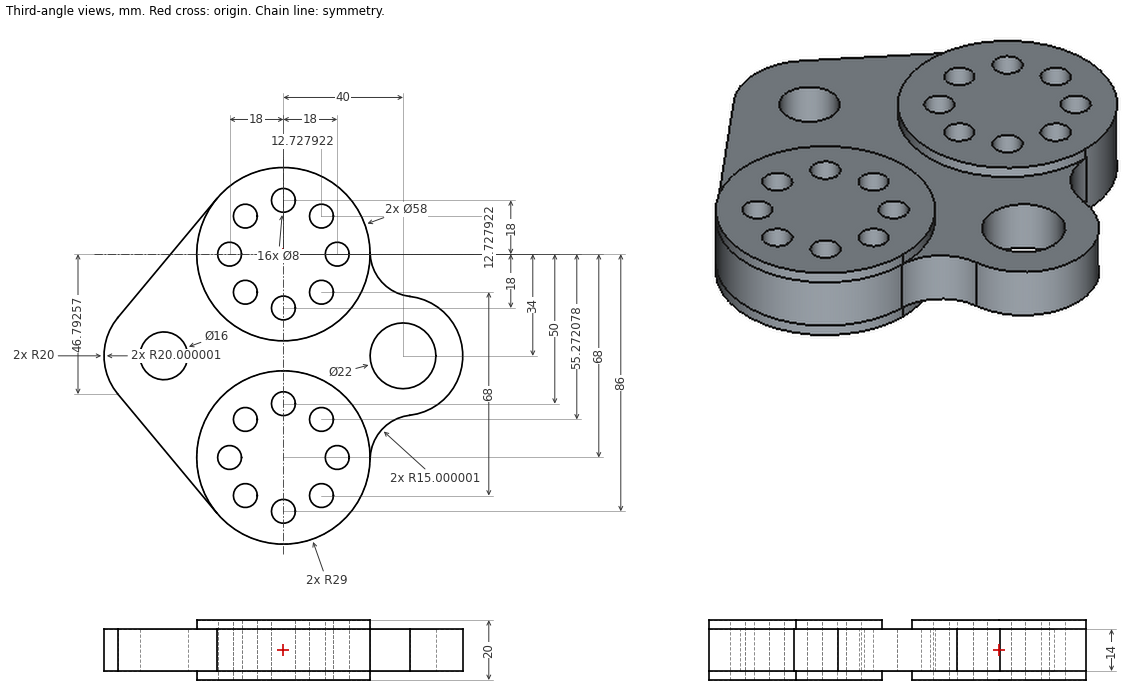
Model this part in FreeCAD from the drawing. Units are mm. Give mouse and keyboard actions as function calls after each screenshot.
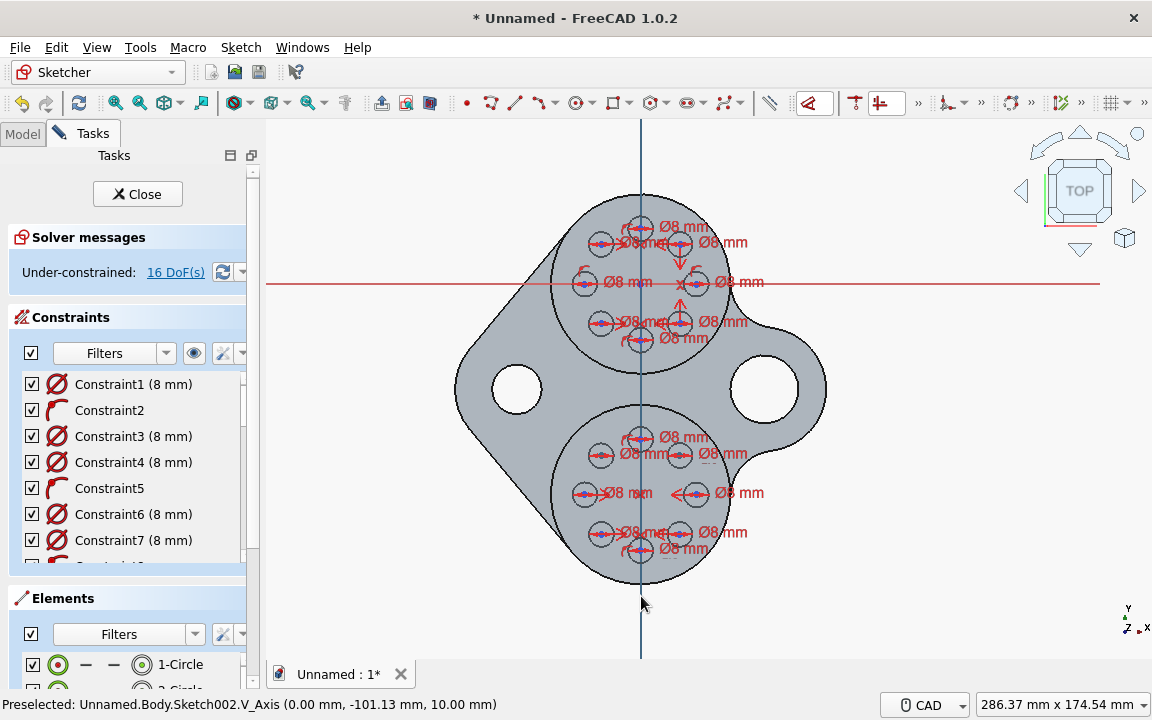
key(s)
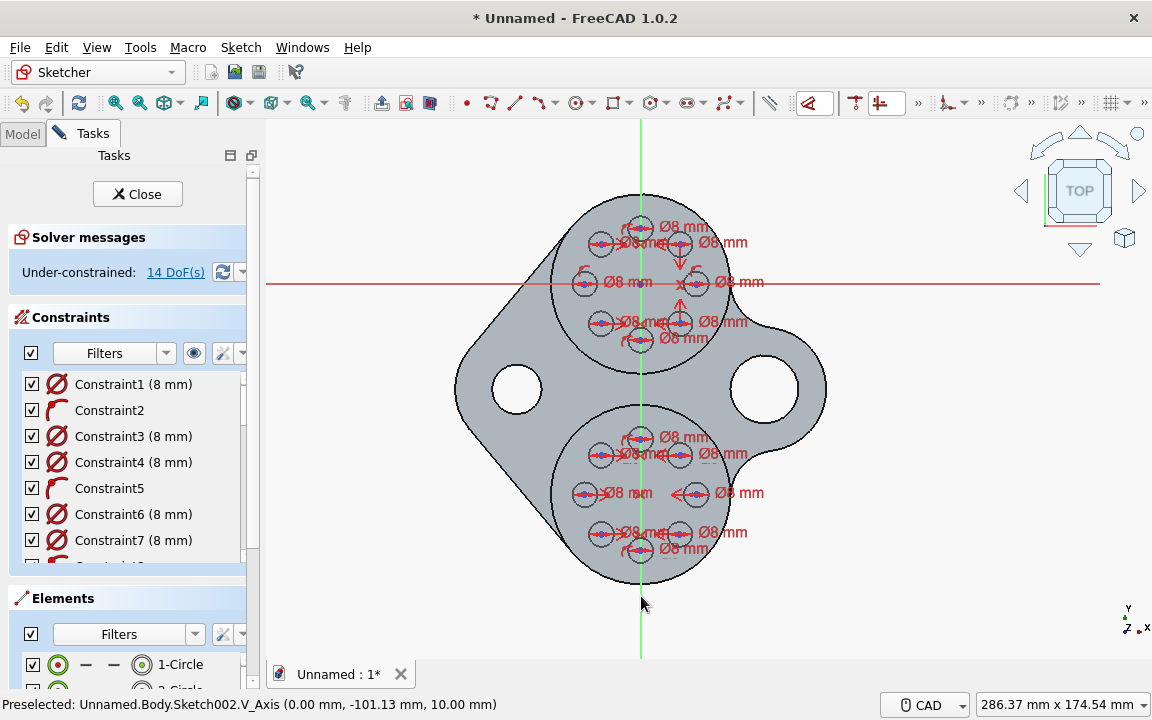
click(641, 229)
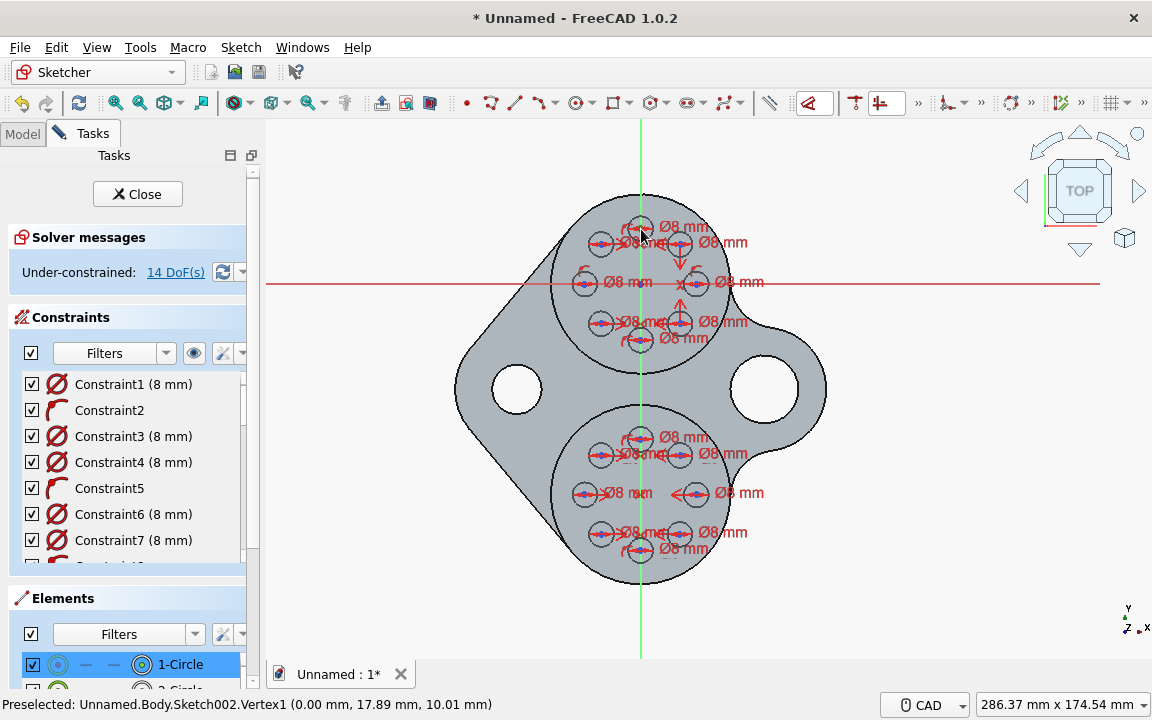
key(i)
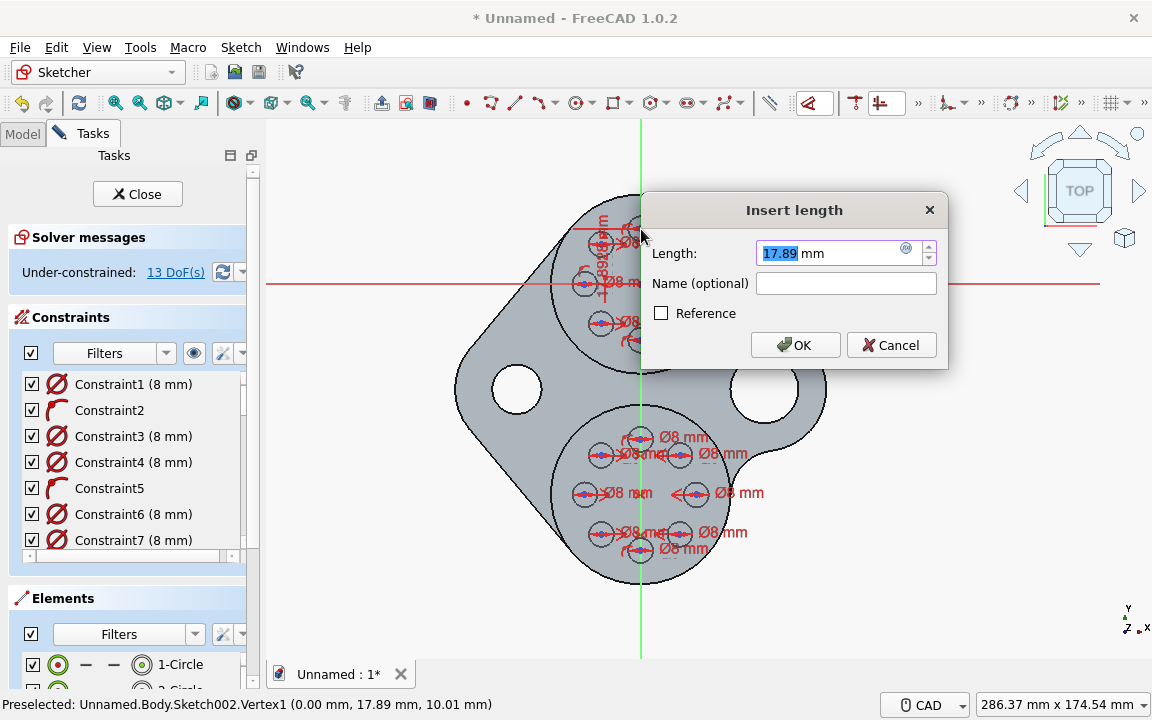
text(18)
key(Return)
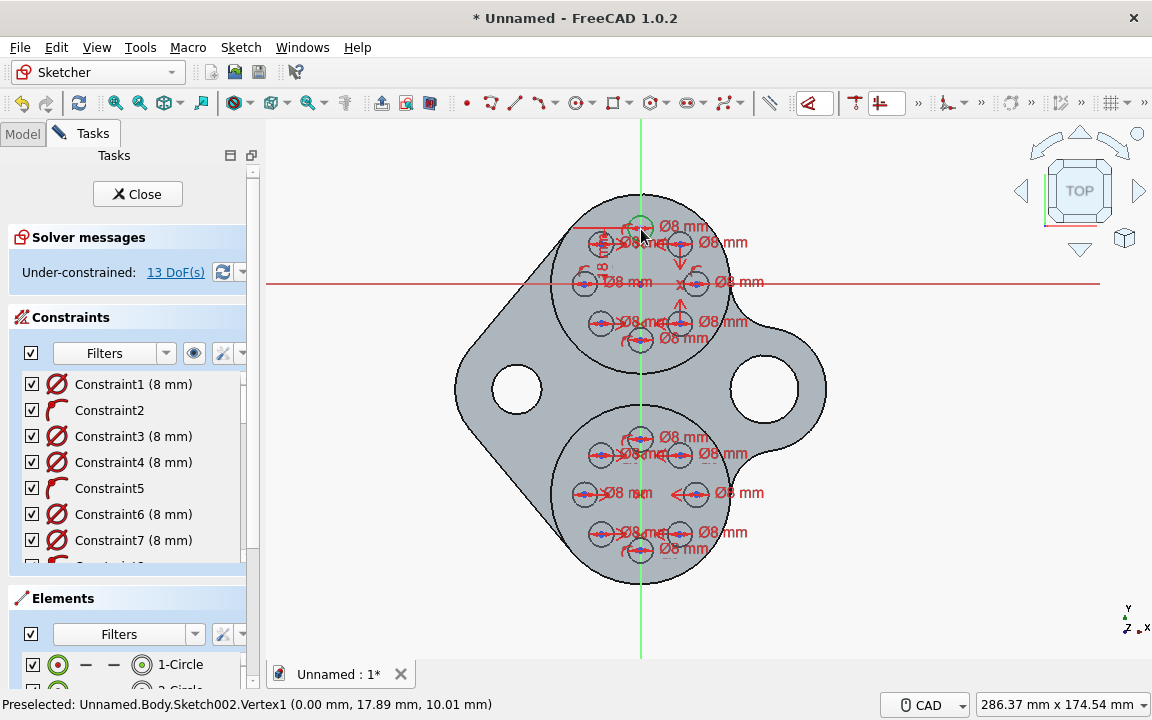
click(696, 284)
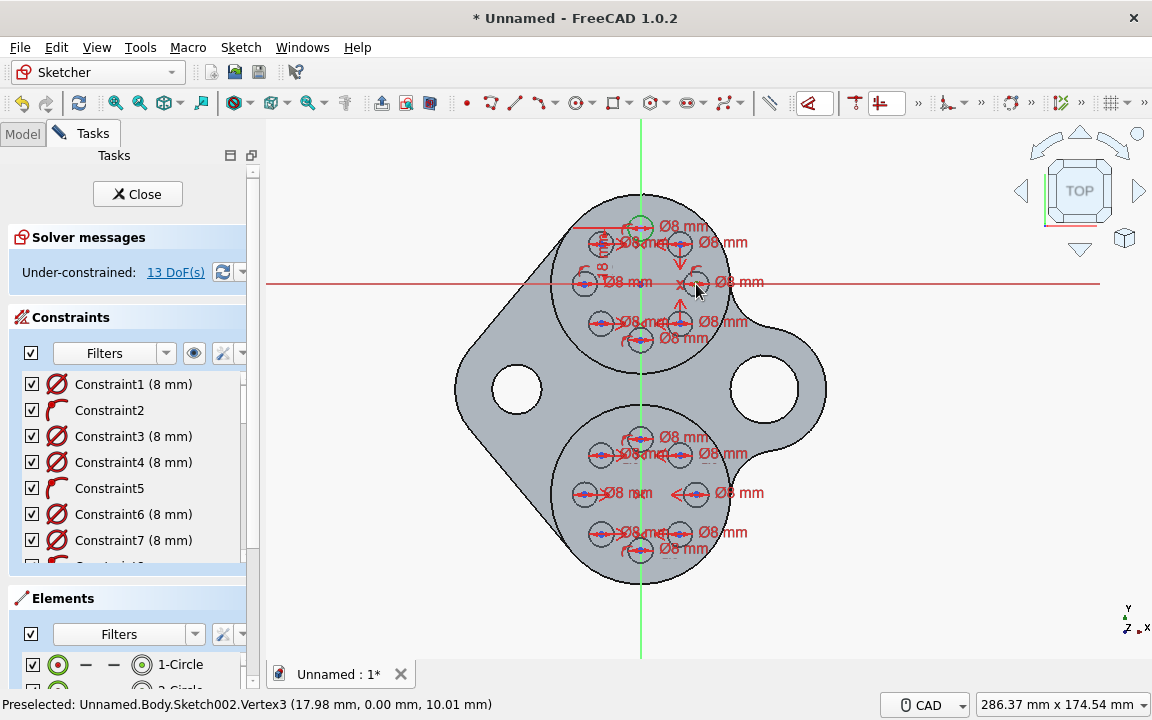
key(l)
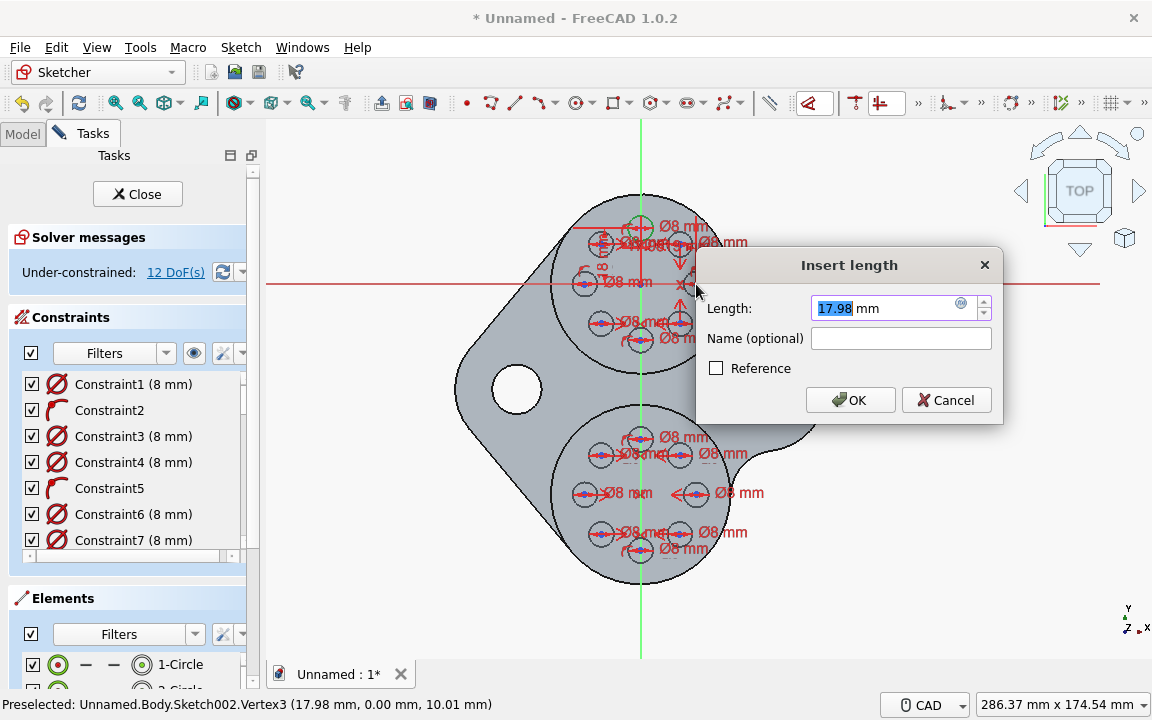
text(18)
key(Return)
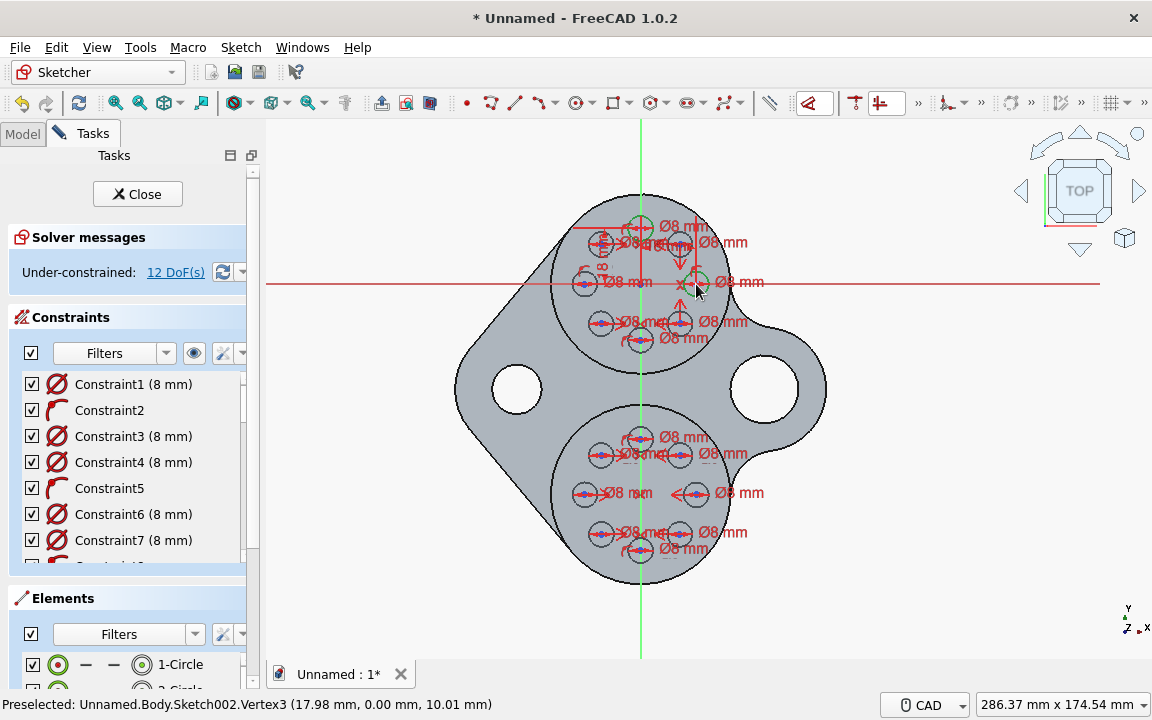
click(641, 340)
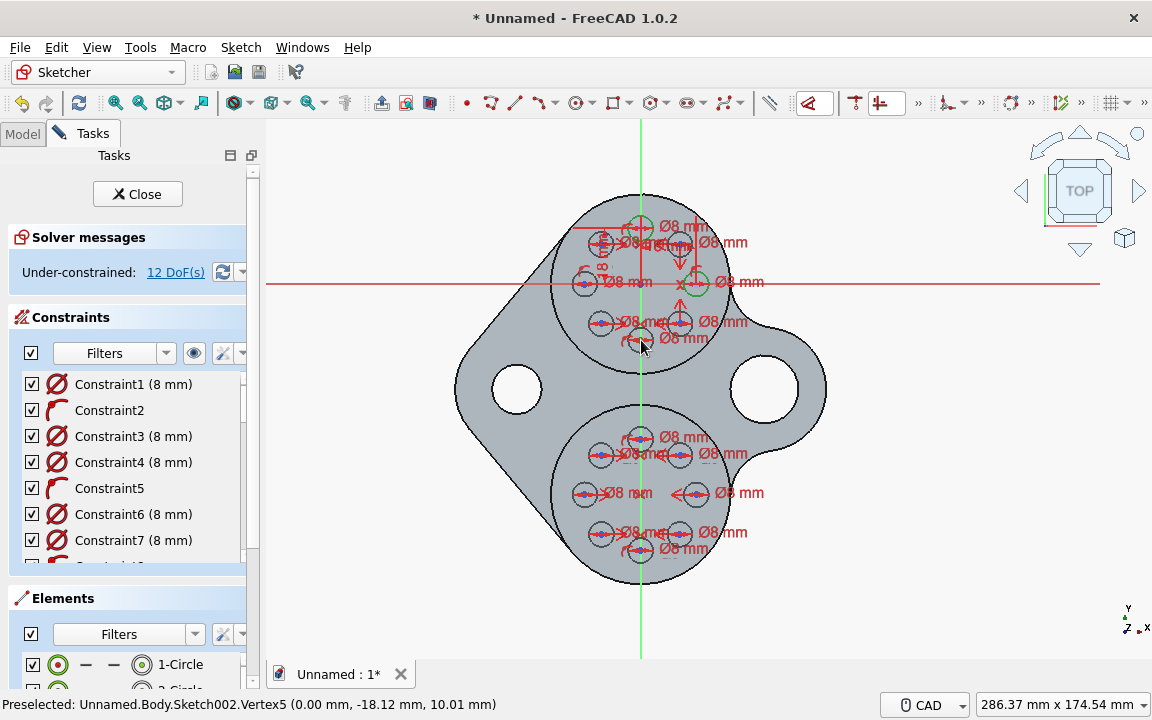
key(i)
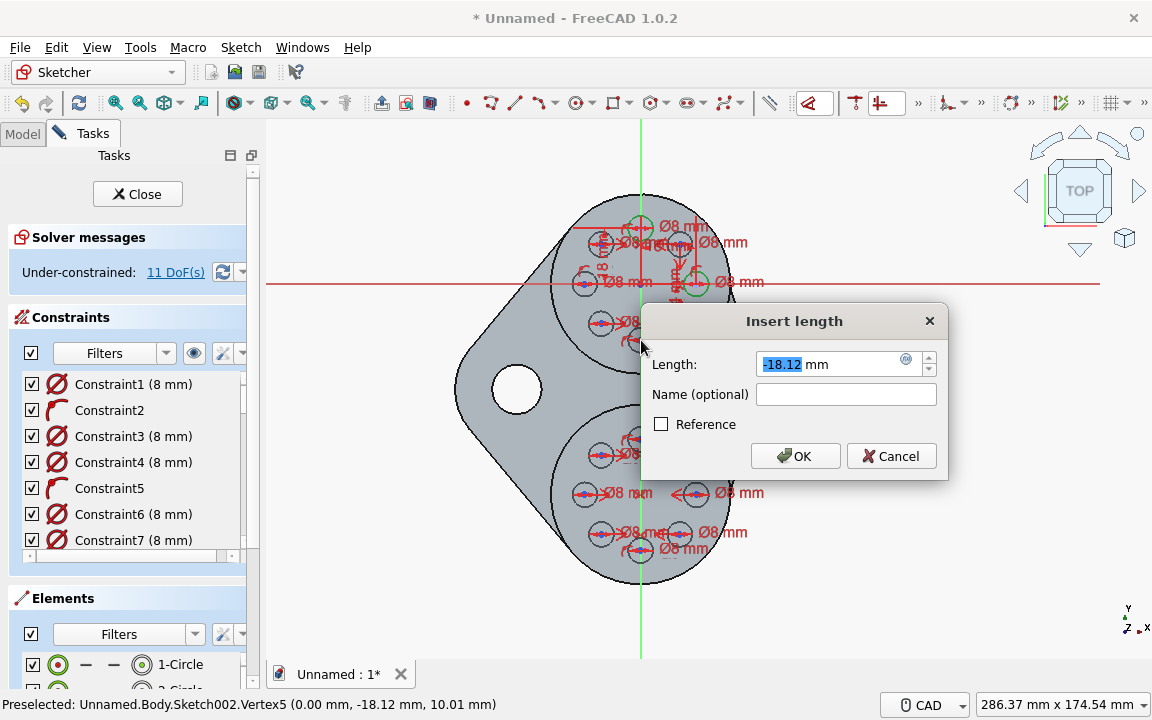
text(-18)
key(Return)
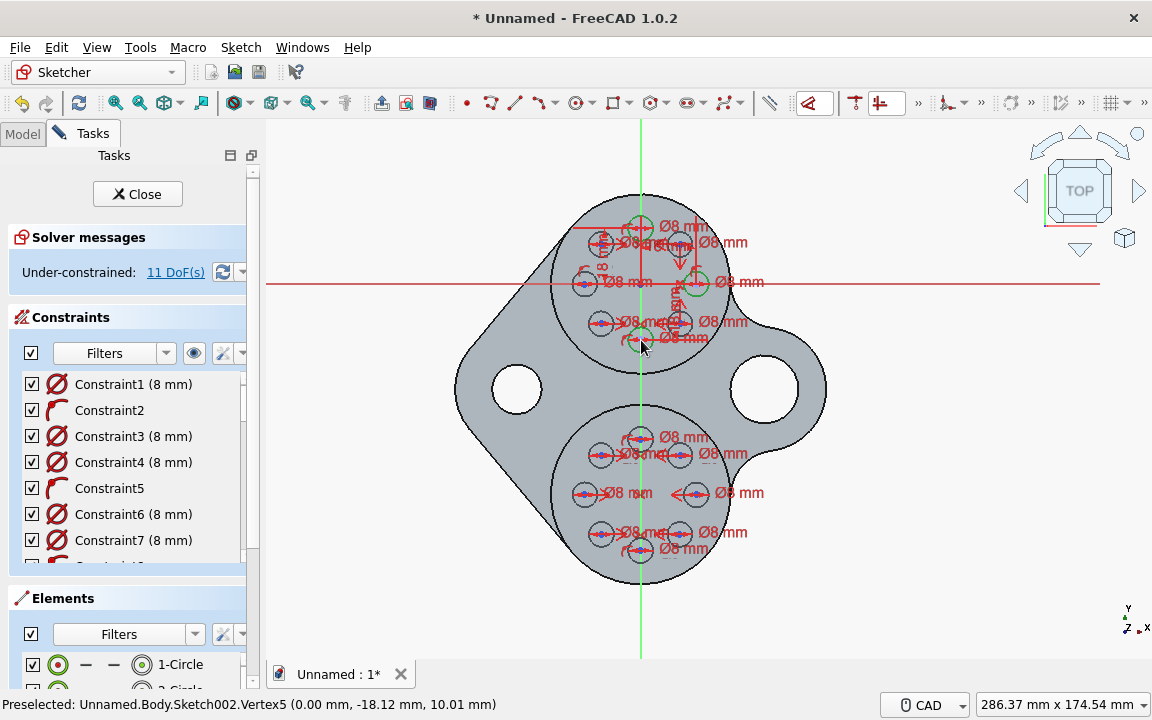
click(585, 284)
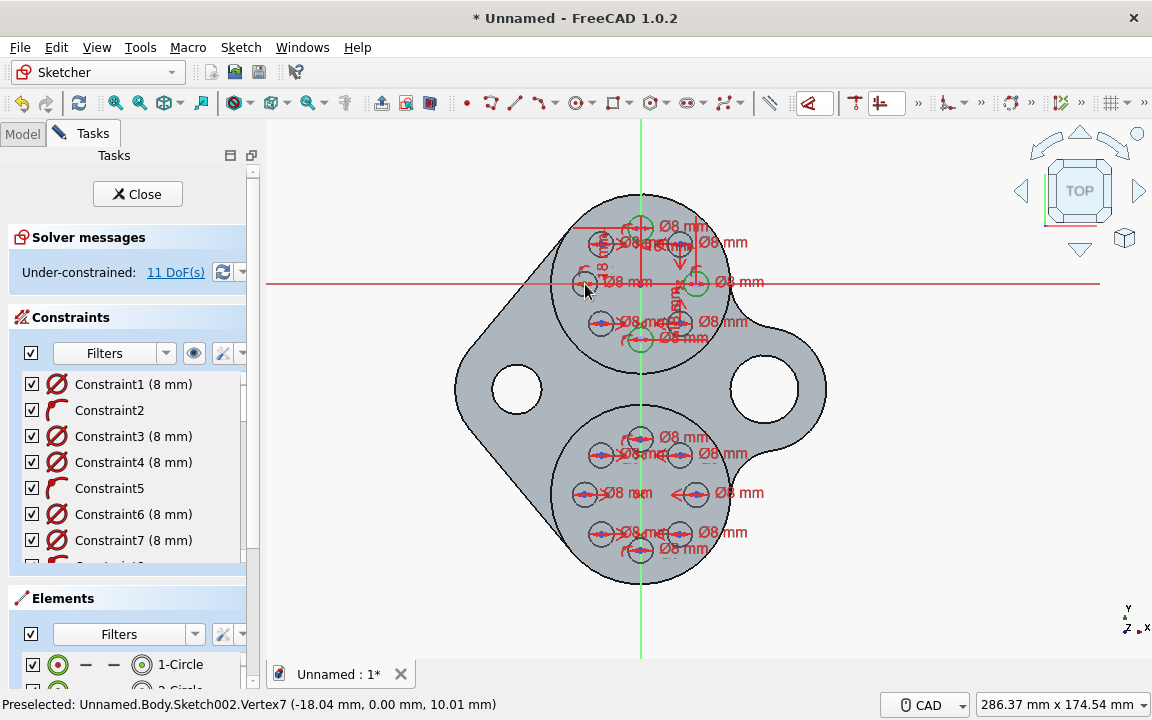
key(l)